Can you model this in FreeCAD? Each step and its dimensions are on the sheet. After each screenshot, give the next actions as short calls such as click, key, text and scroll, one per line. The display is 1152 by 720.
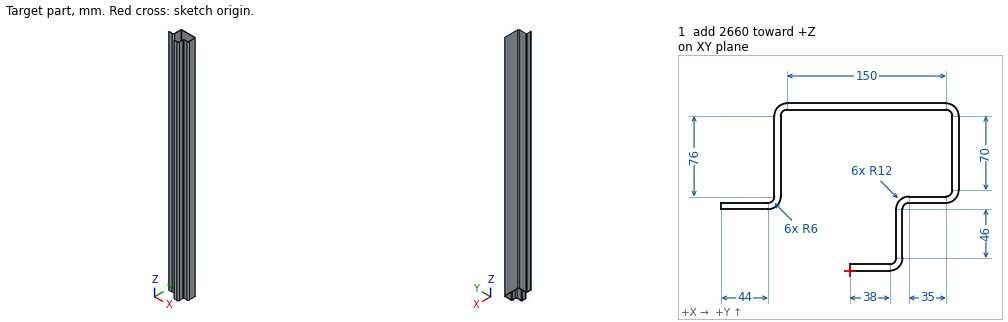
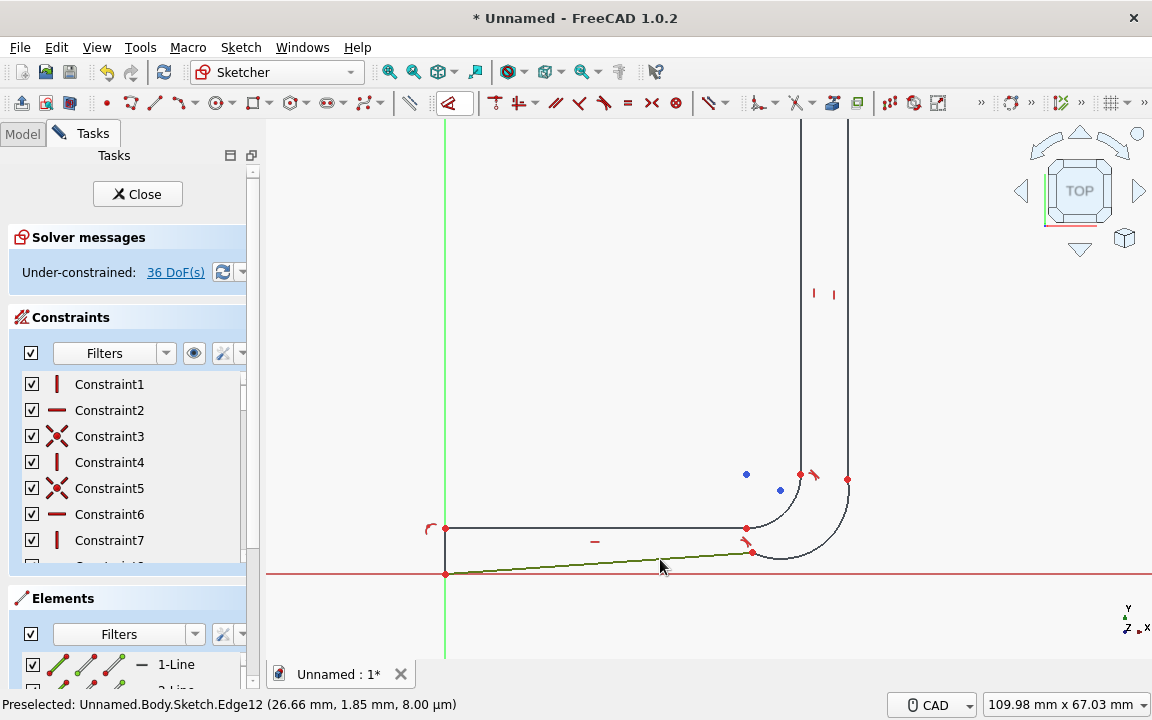
click(796, 557)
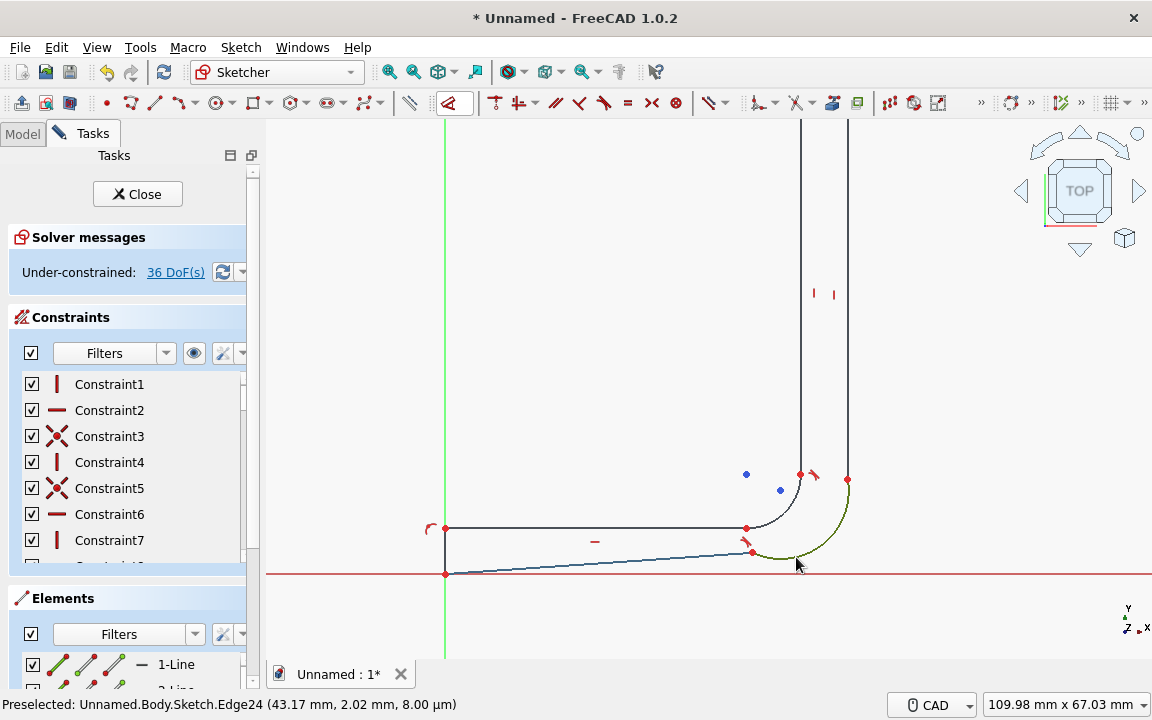
key(t)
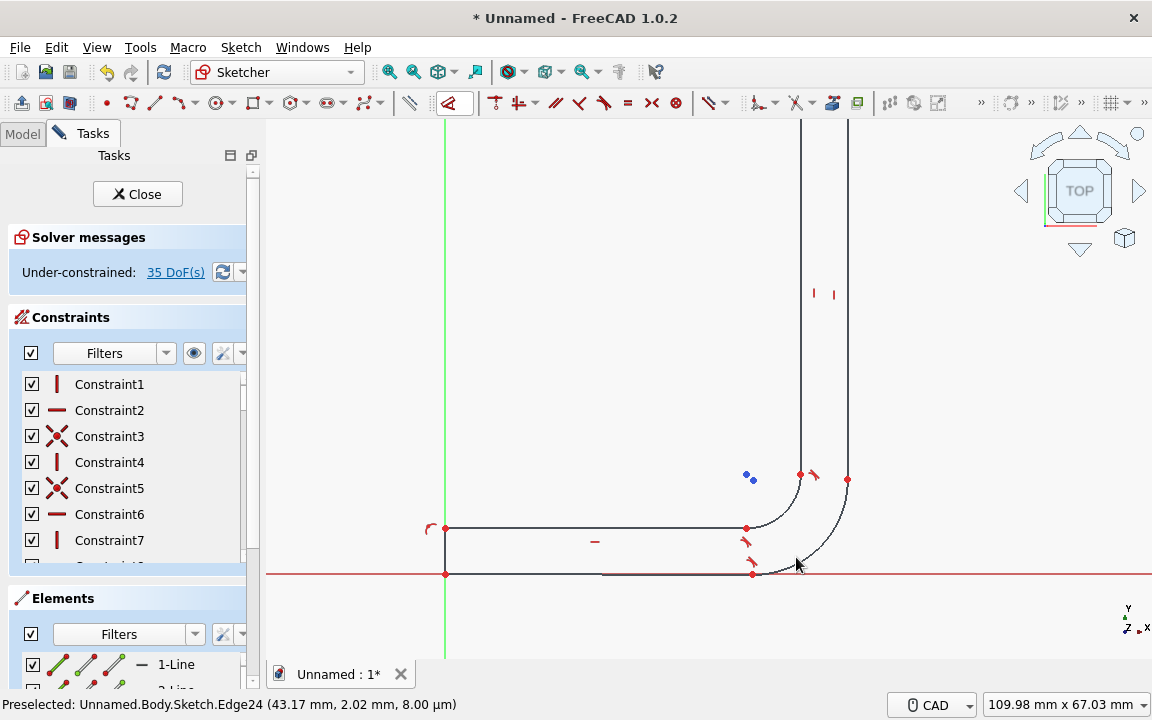
scroll(728, 537, down, 7)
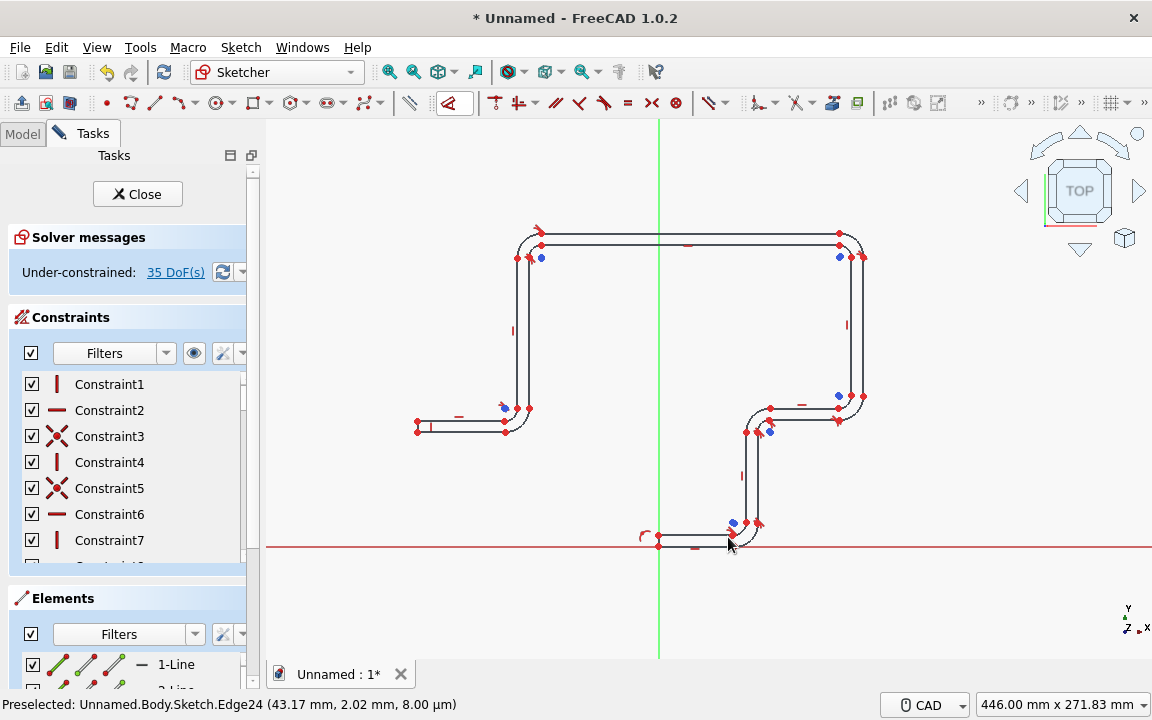
click(758, 496)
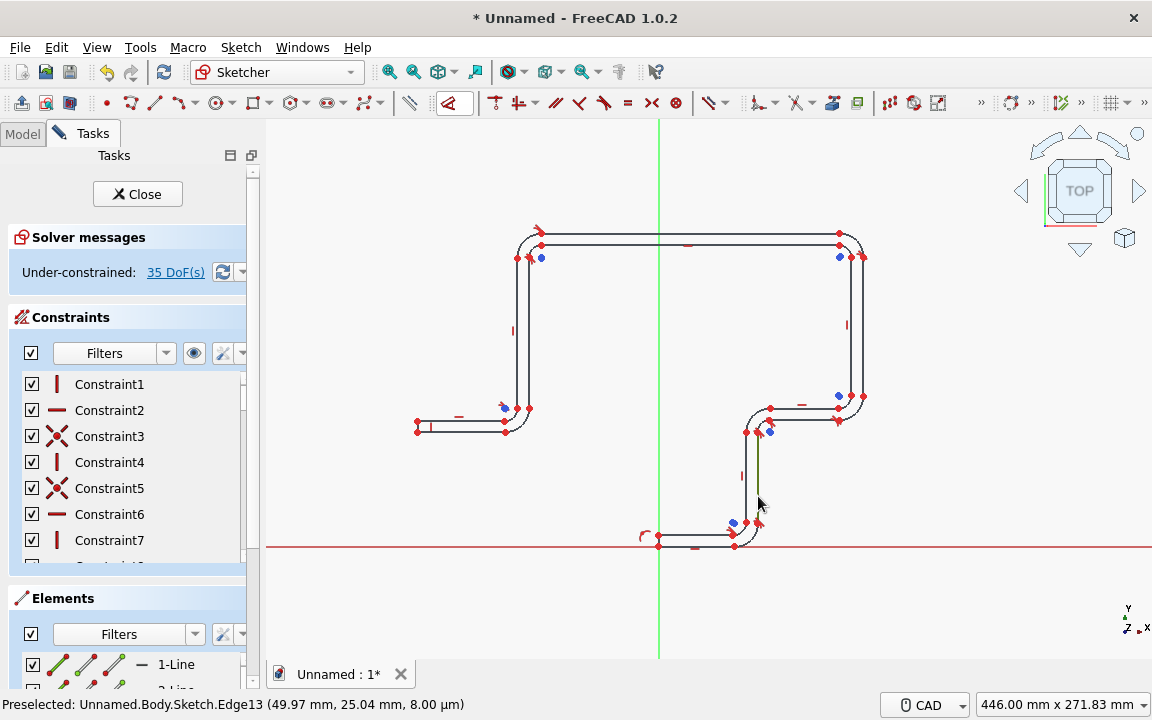
scroll(745, 544, up, 2)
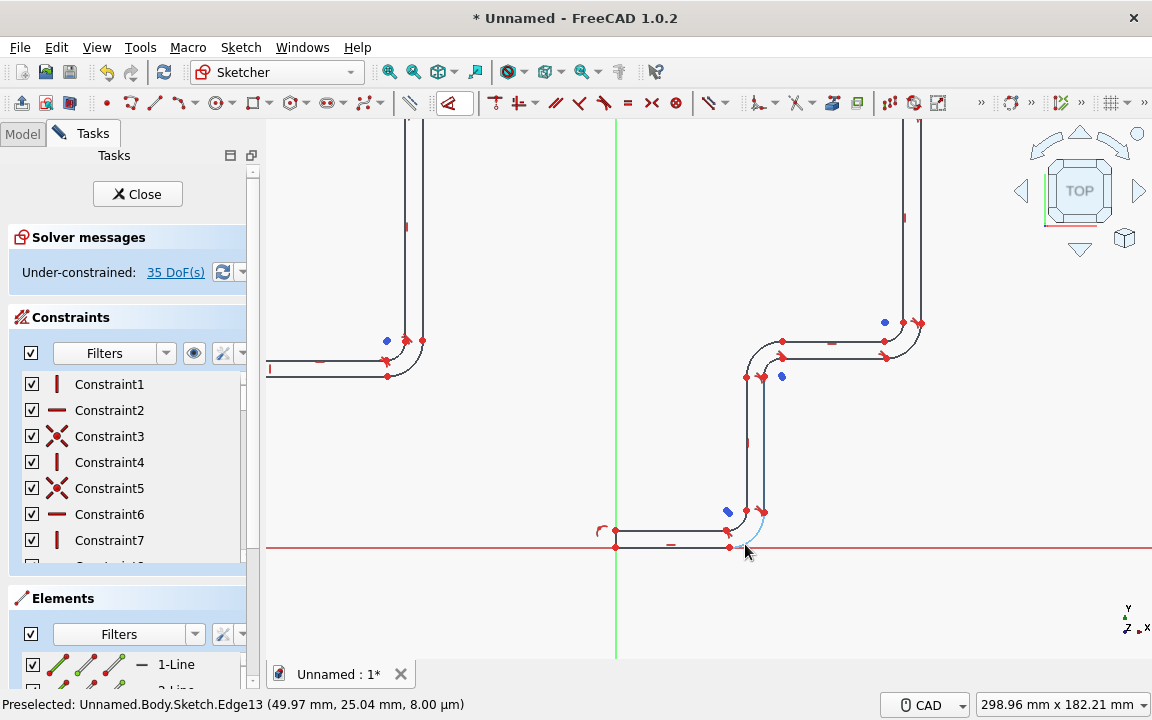
click(745, 544)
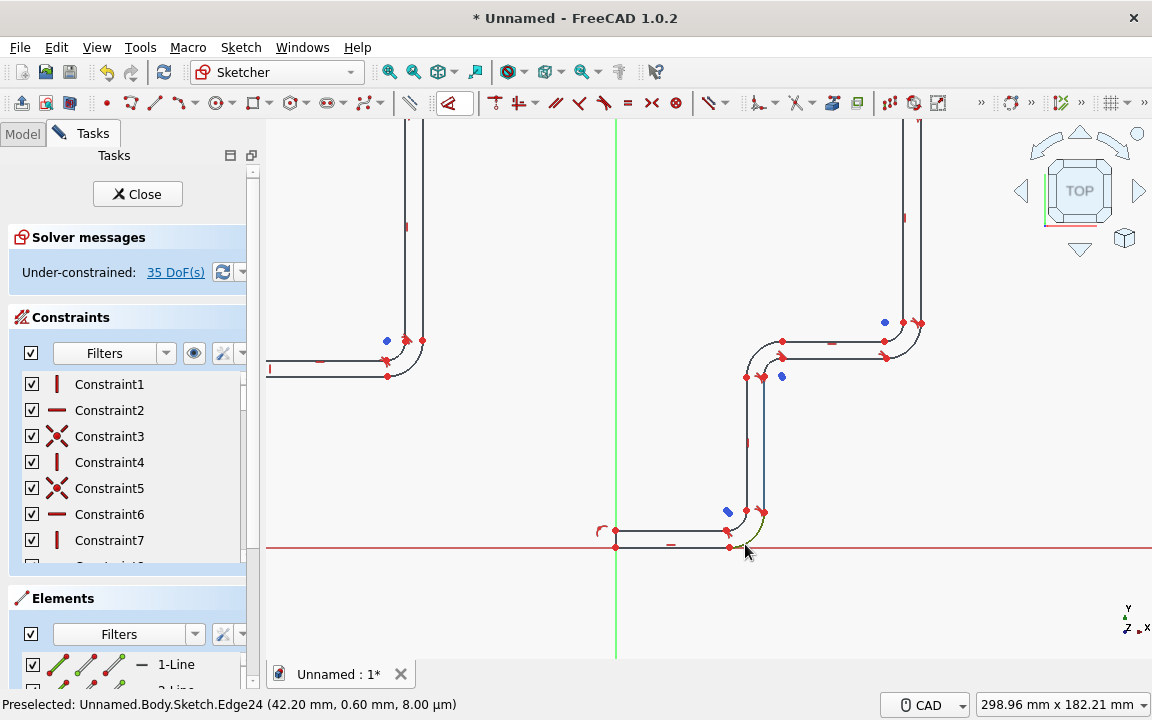
click(604, 104)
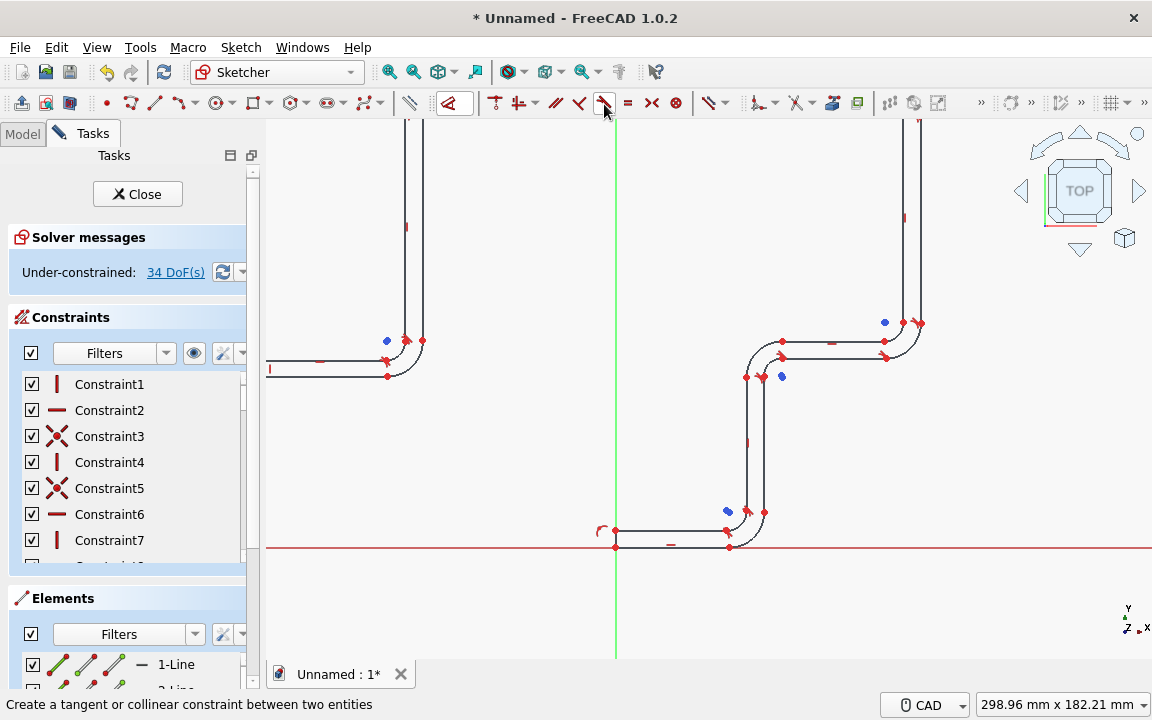
click(764, 472)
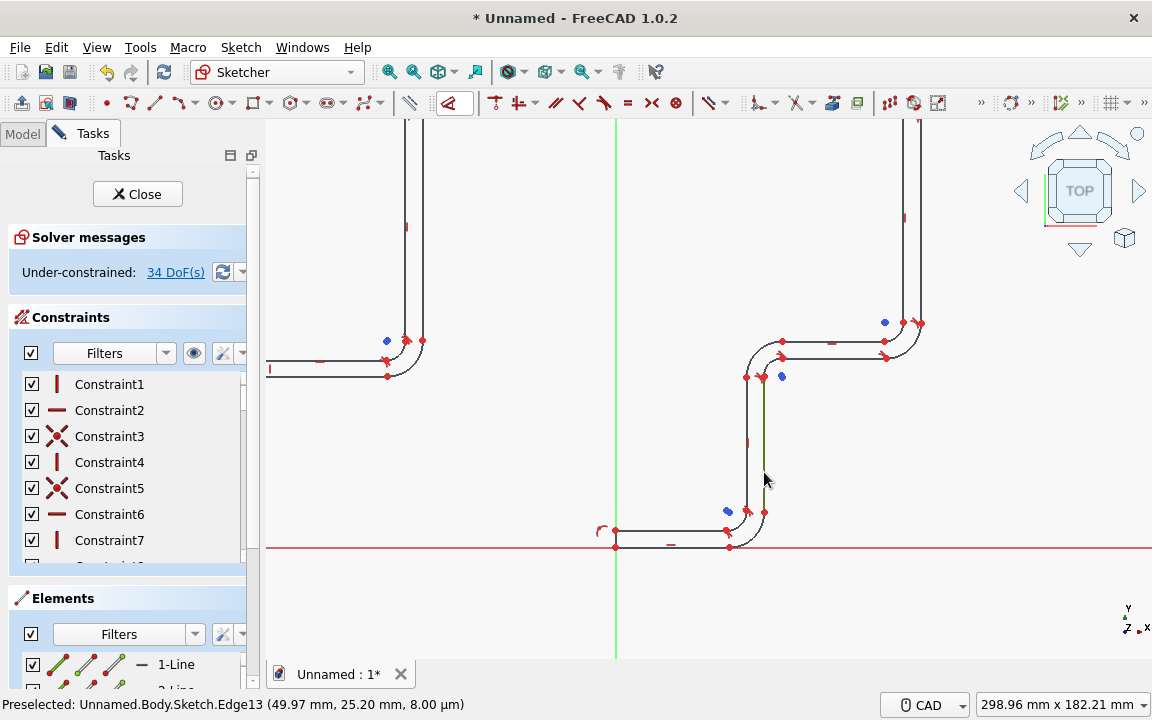
click(769, 364)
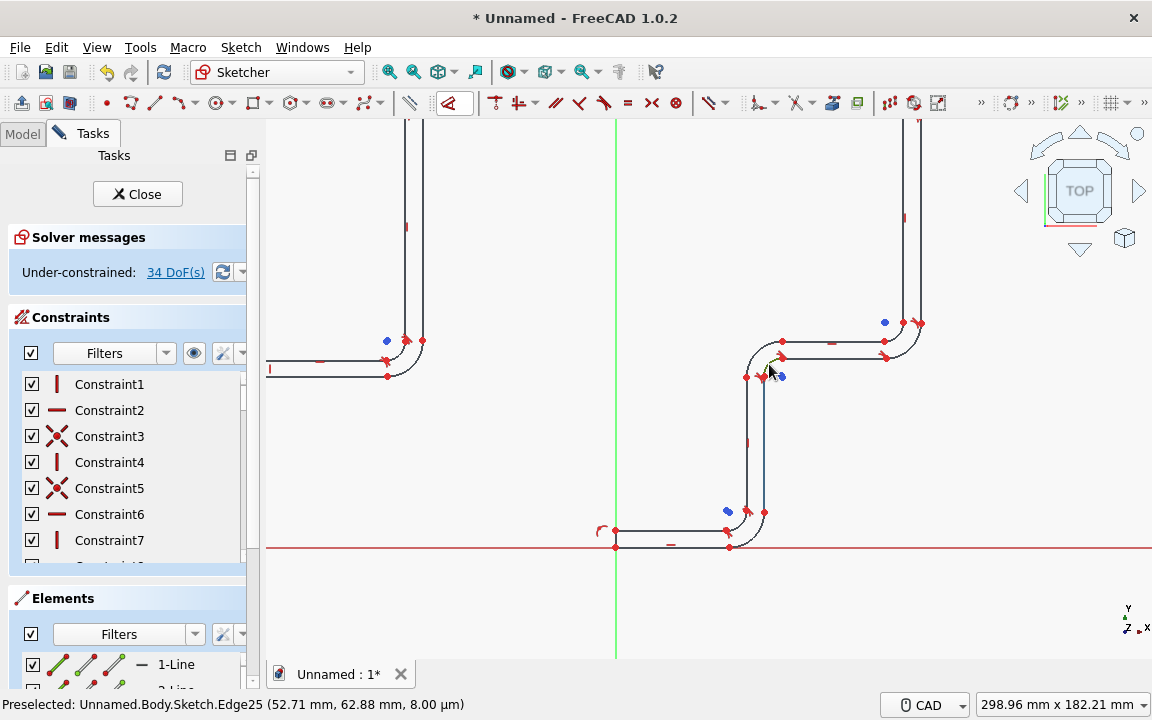
key(t)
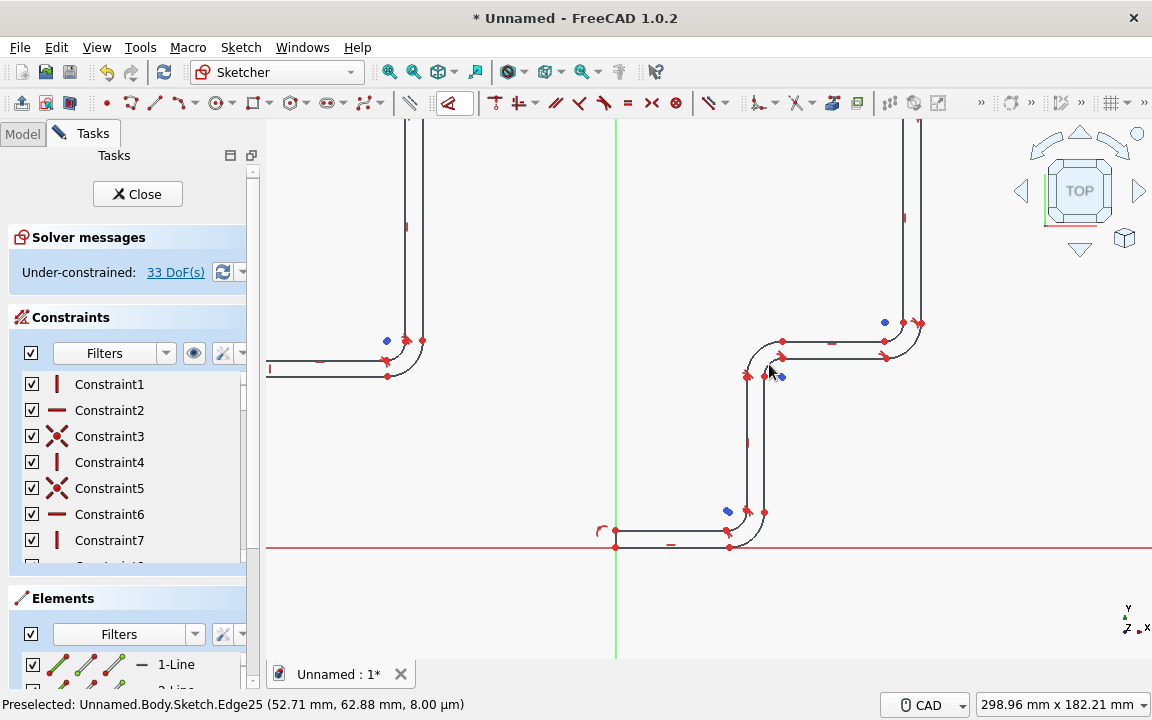
click(813, 359)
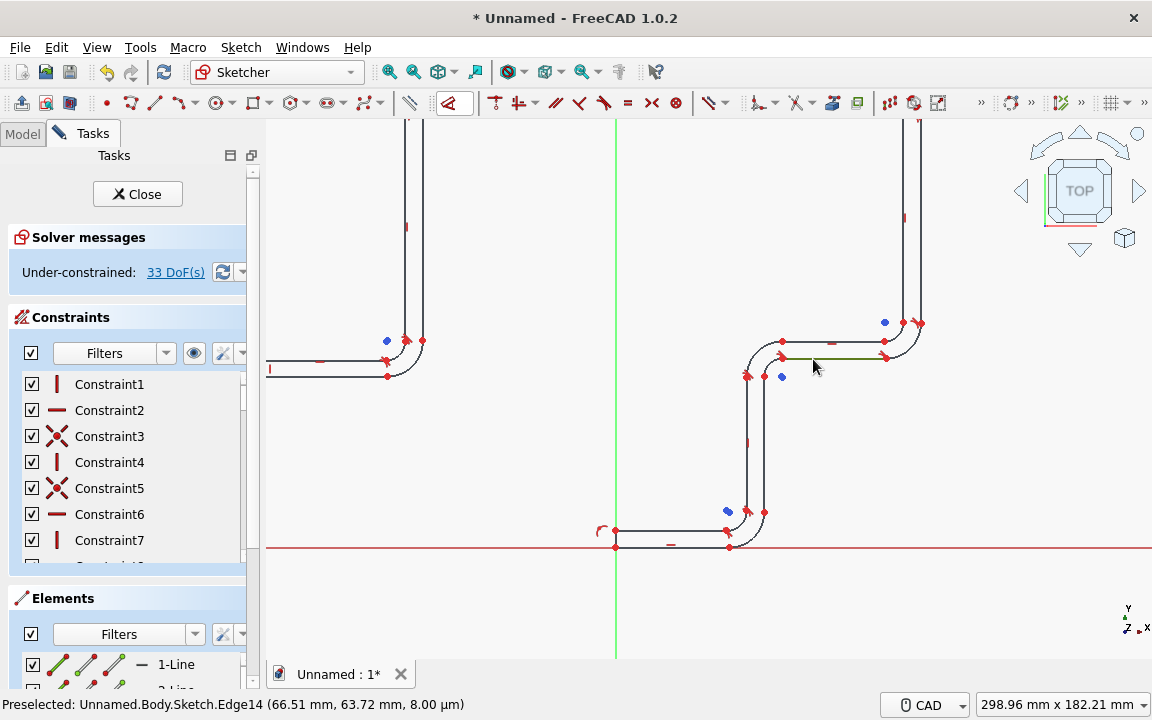
click(769, 364)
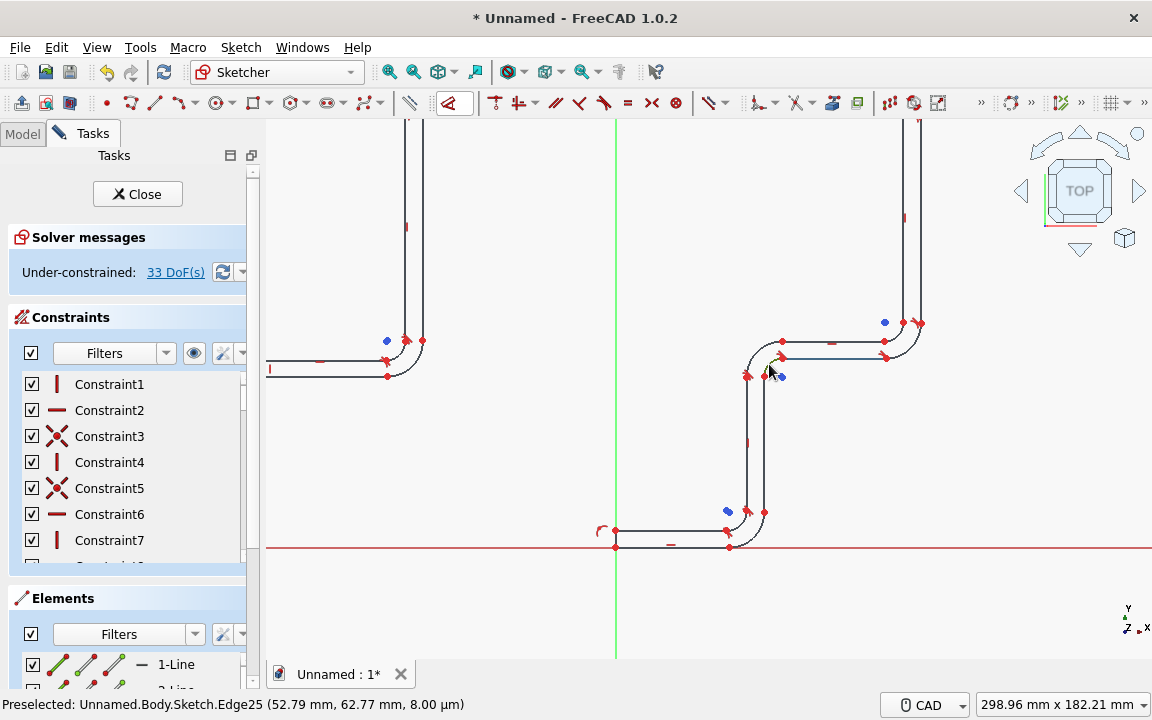
click(604, 104)